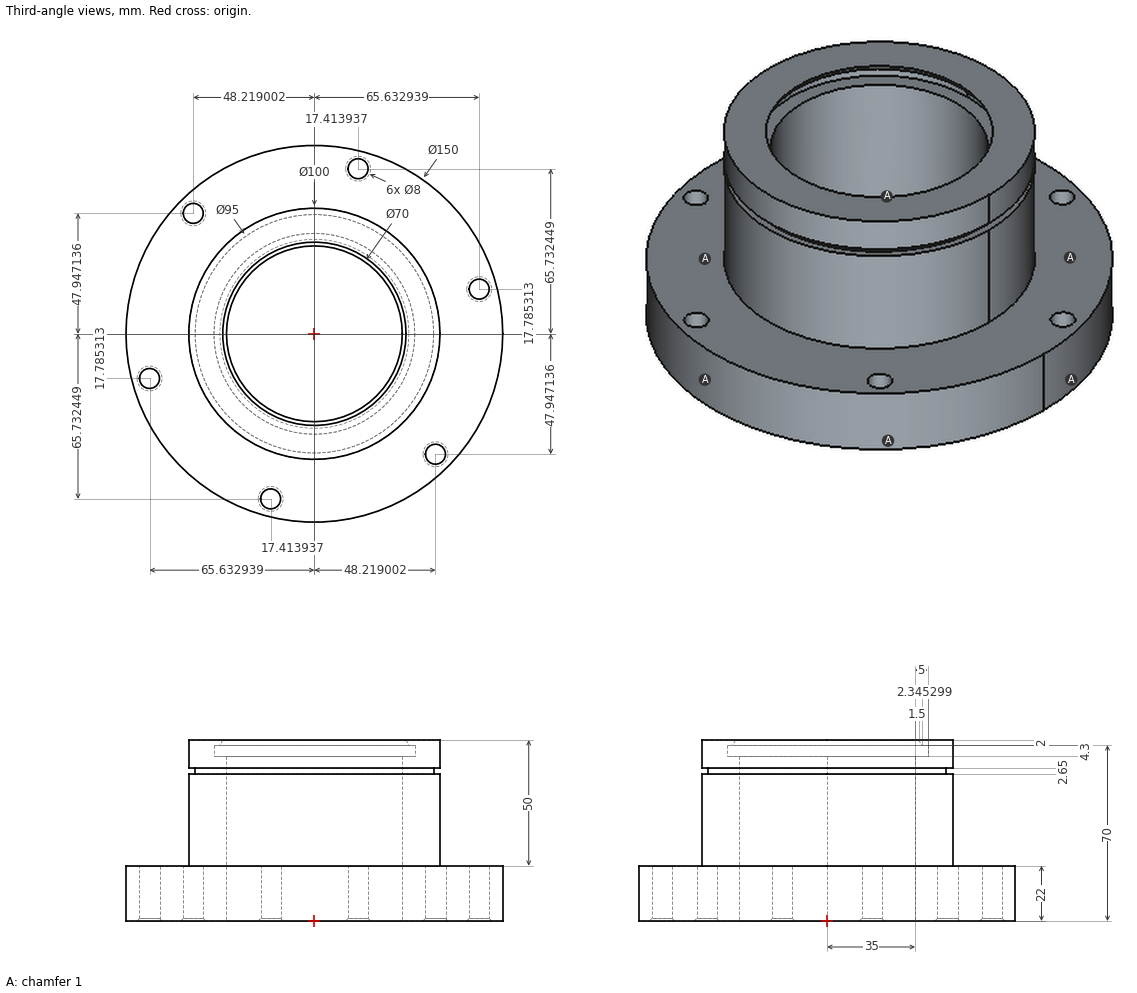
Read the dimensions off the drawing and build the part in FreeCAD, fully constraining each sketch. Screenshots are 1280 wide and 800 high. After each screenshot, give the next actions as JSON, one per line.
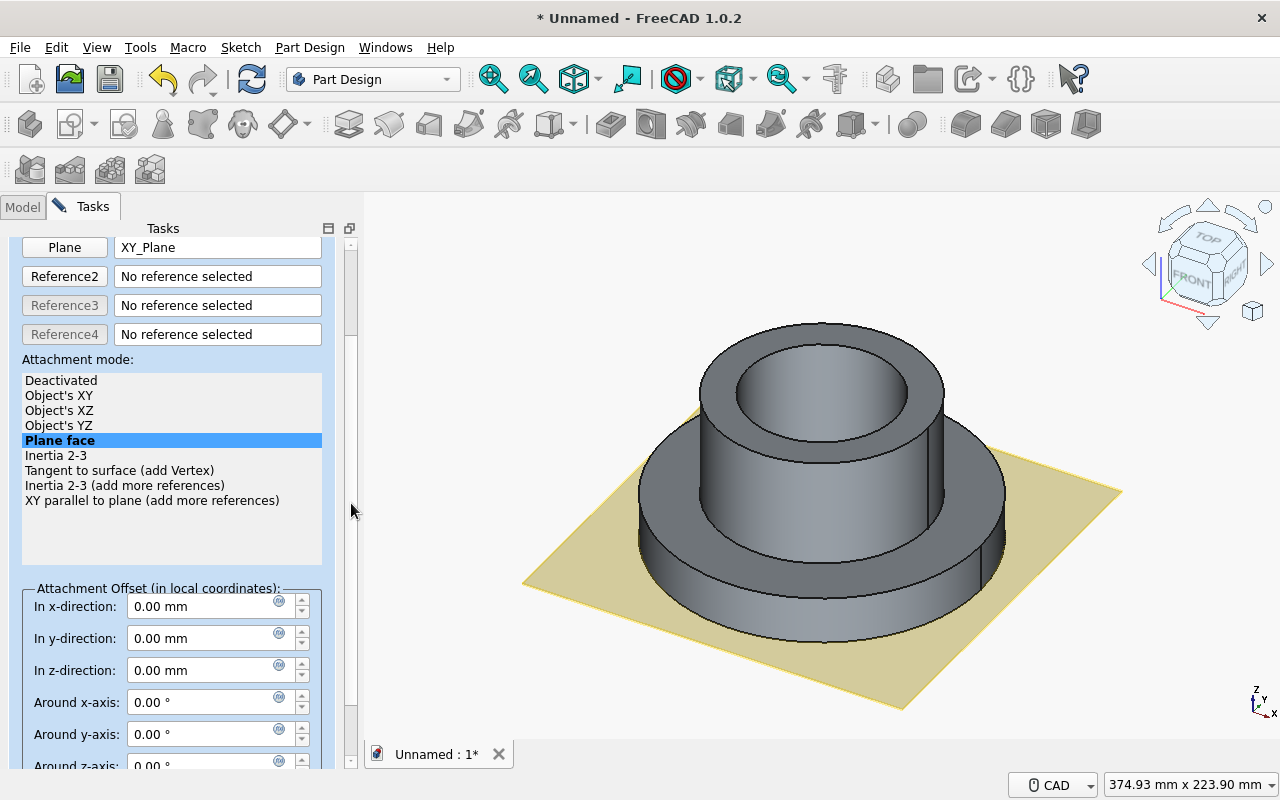
{"action": "triple_click", "coordinate": [210, 670]}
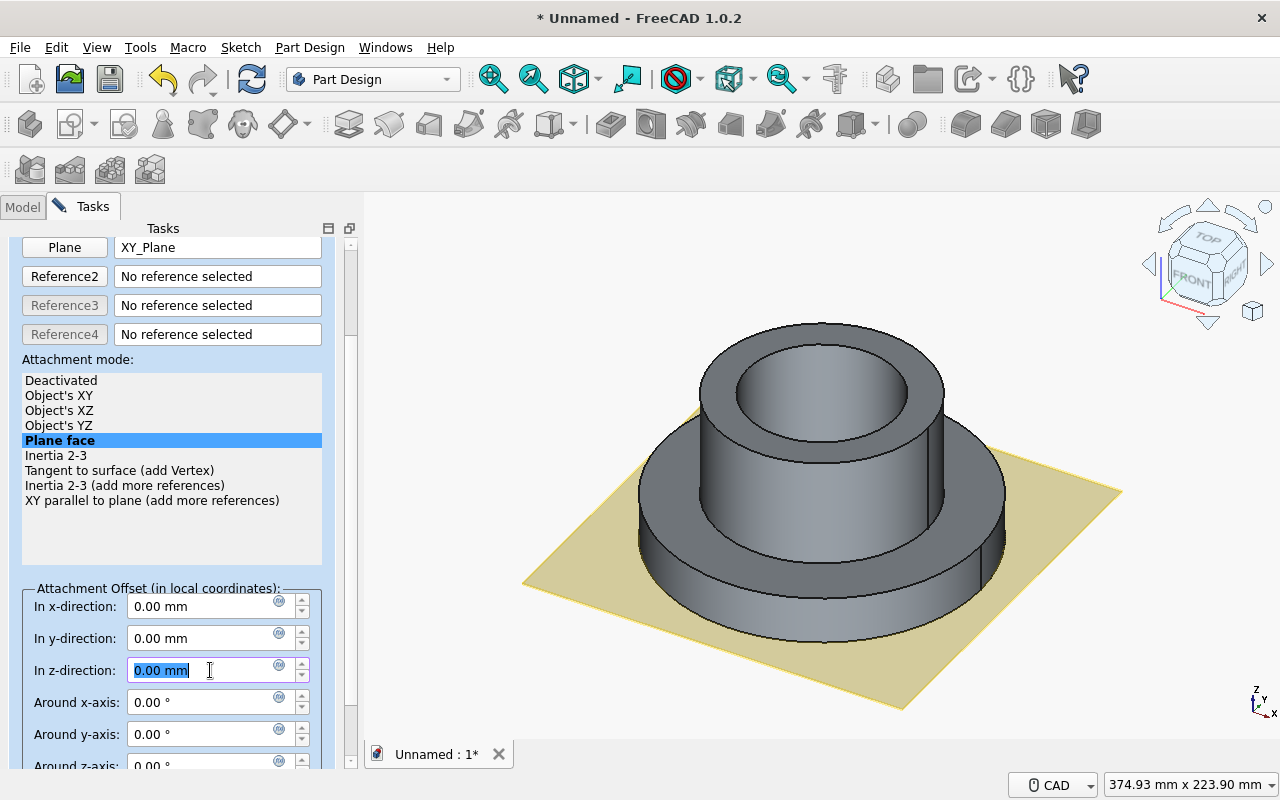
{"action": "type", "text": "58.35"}
{"action": "key", "text": "Tab"}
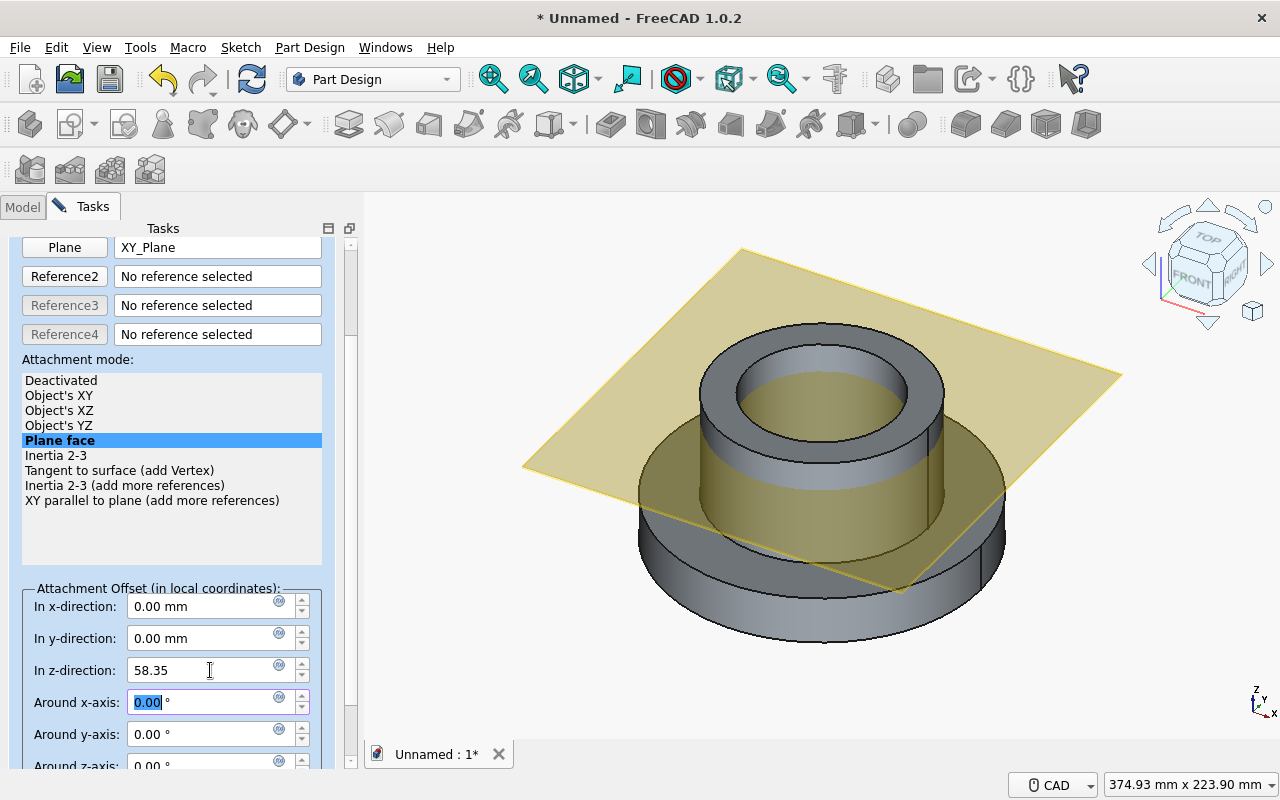
{"action": "scroll", "coordinate": [351, 503], "scroll_direction": "up", "scroll_amount": 3}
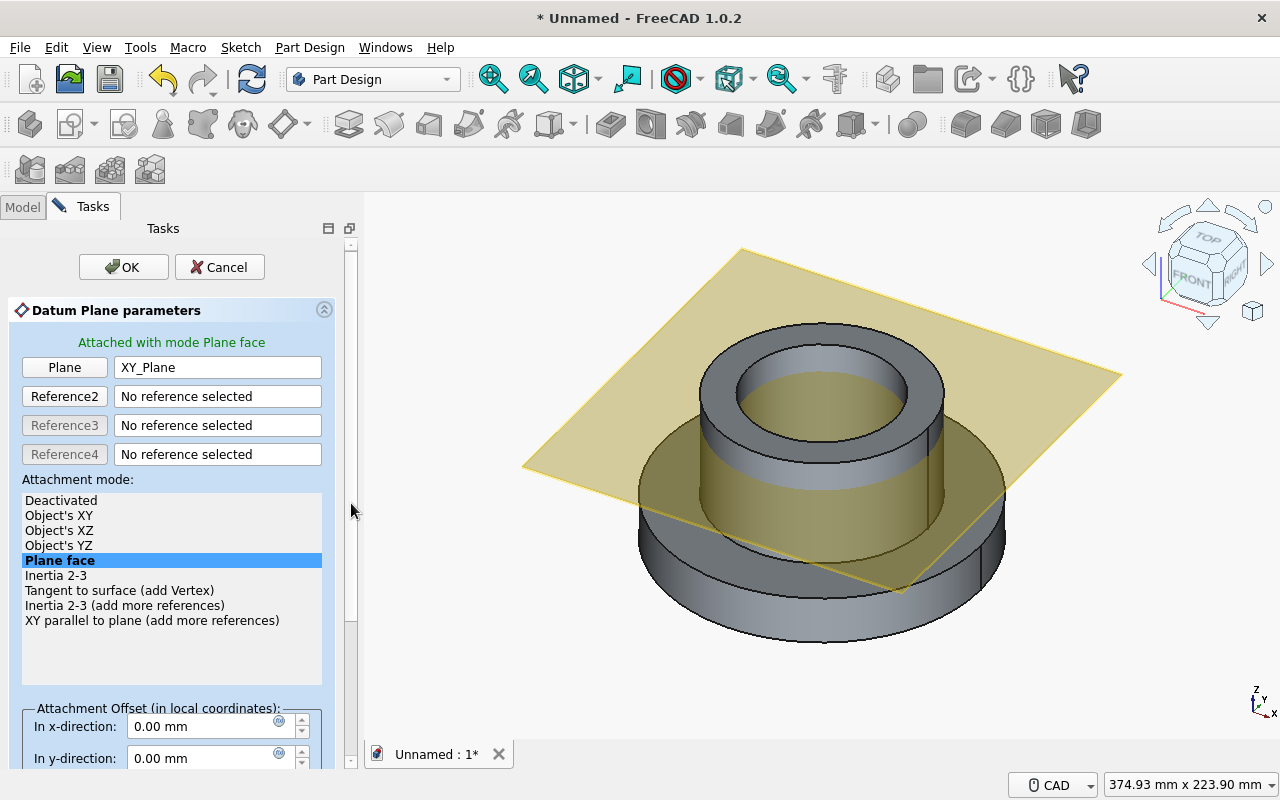
{"action": "left_click", "coordinate": [124, 267]}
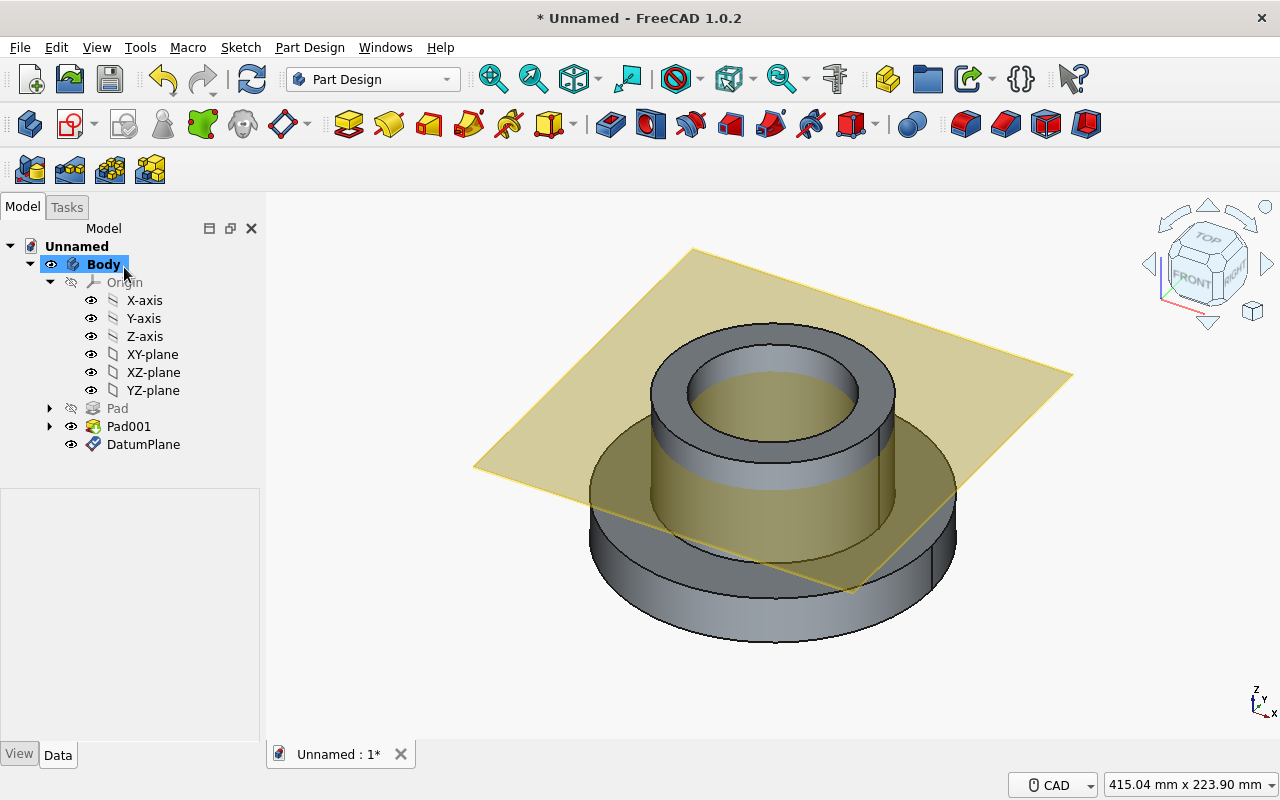
{"action": "left_click", "coordinate": [116, 444]}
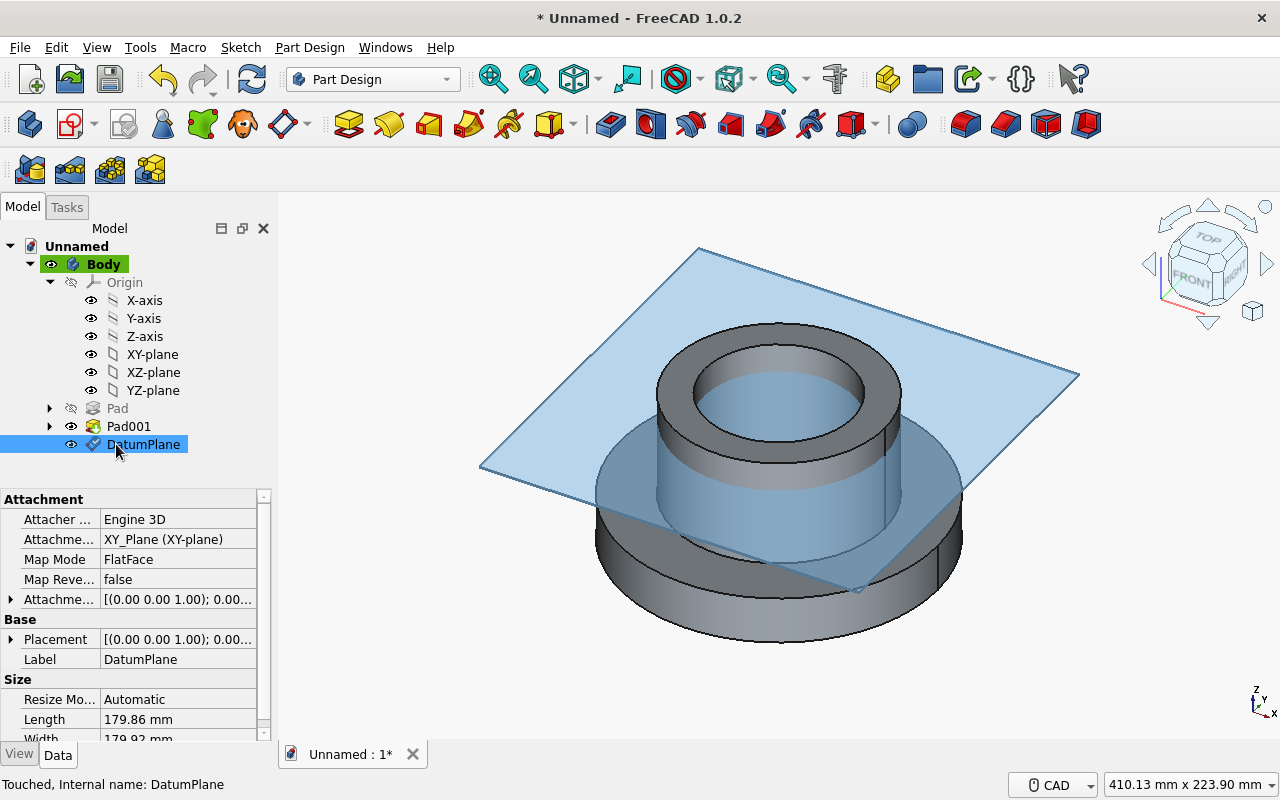
{"action": "left_click", "coordinate": [70, 124]}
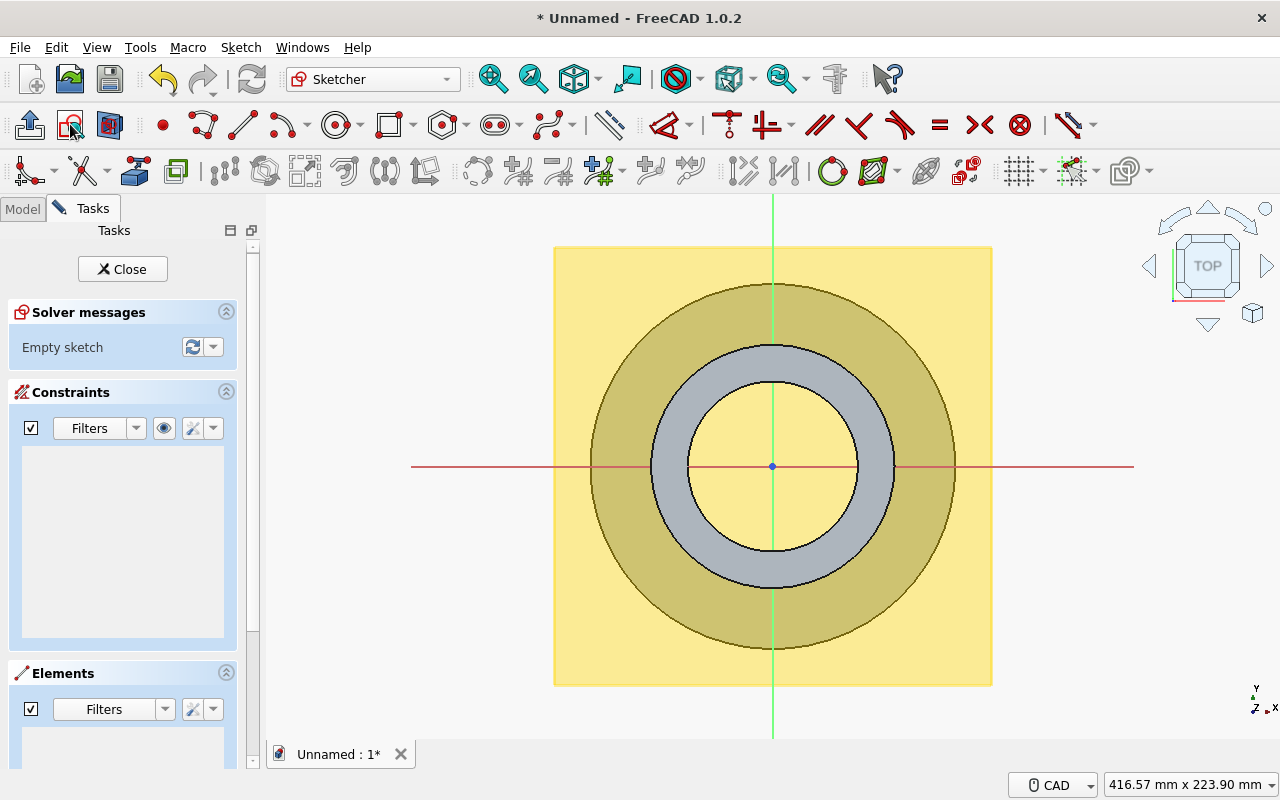
{"action": "left_click", "coordinate": [110, 126]}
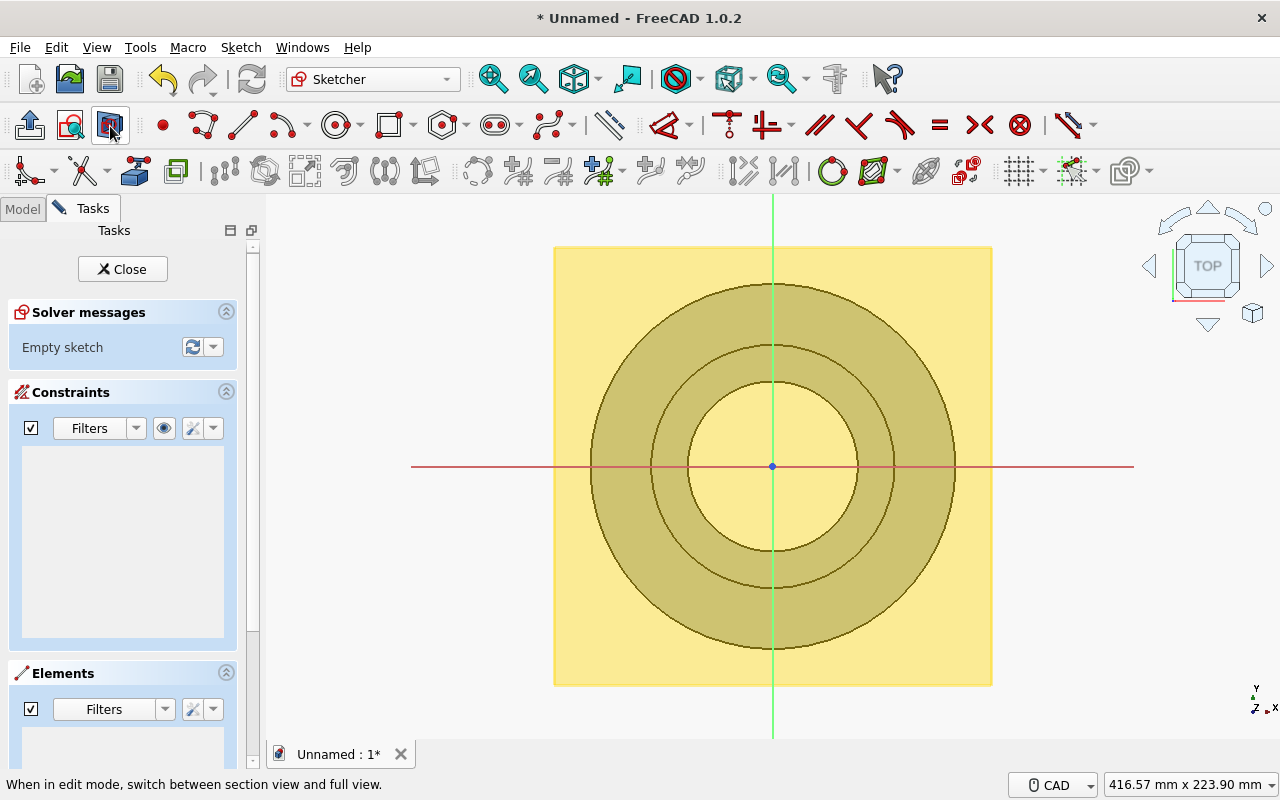
{"action": "scroll", "coordinate": [912, 467], "scroll_direction": "up", "scroll_amount": 2}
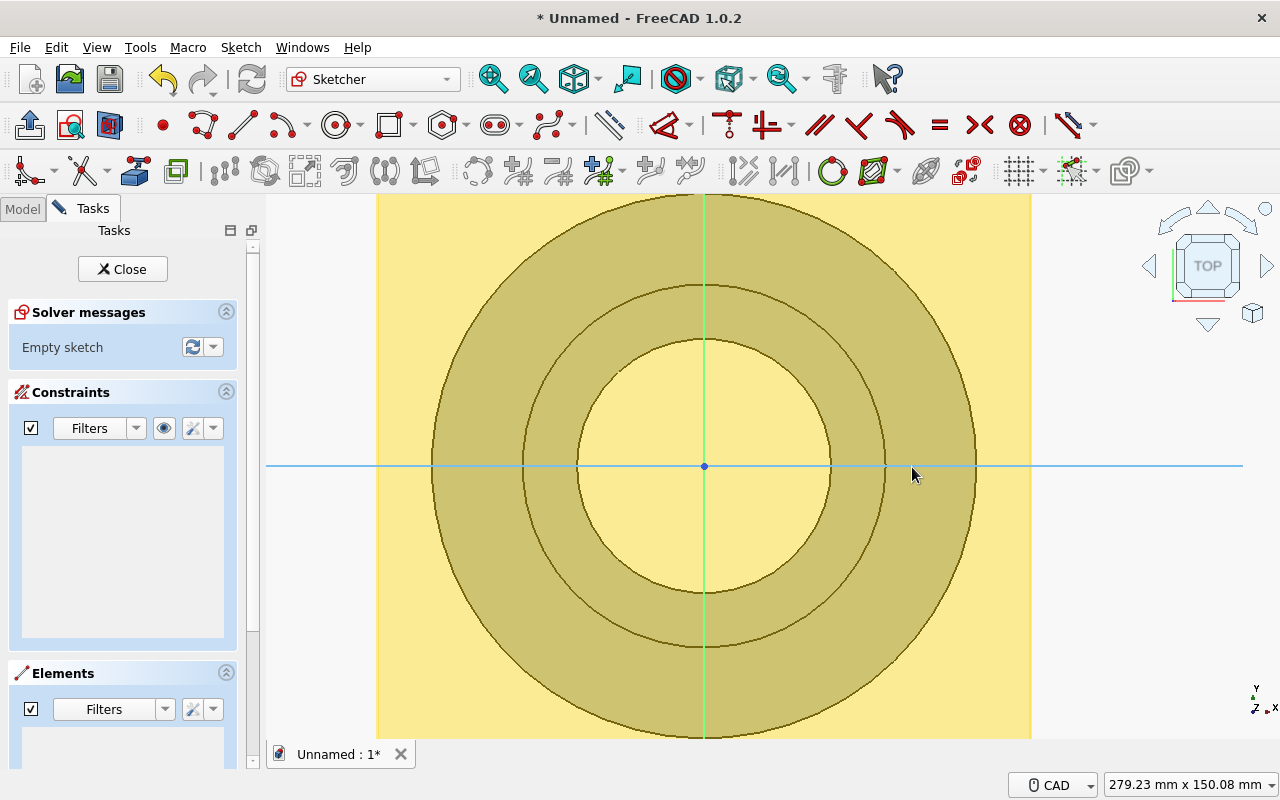
{"action": "left_click", "coordinate": [336, 126]}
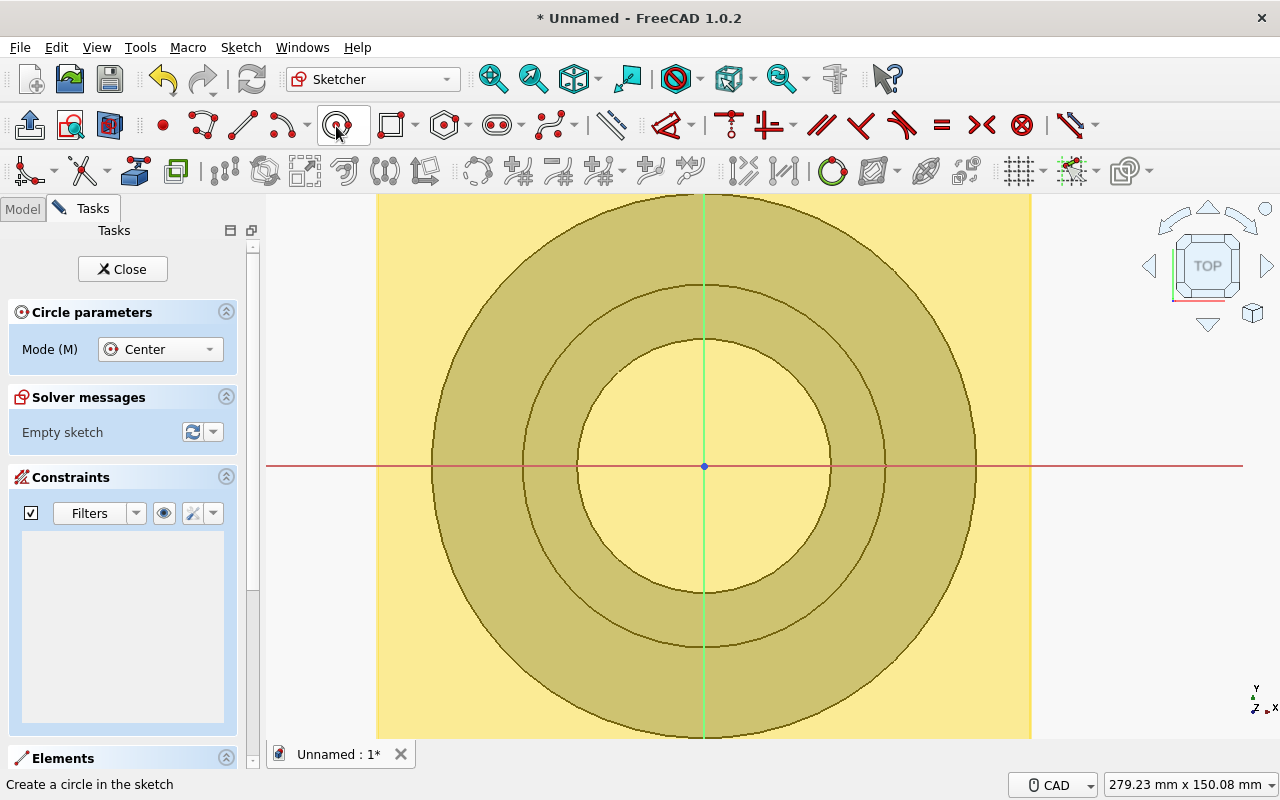
{"action": "left_click", "coordinate": [704, 466]}
{"action": "left_click", "coordinate": [832, 338]}